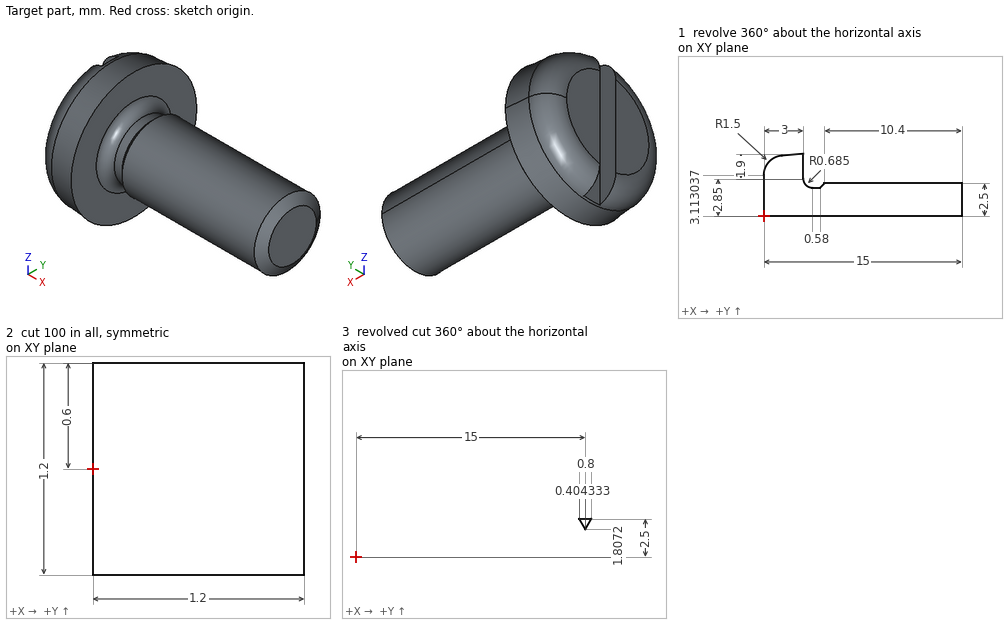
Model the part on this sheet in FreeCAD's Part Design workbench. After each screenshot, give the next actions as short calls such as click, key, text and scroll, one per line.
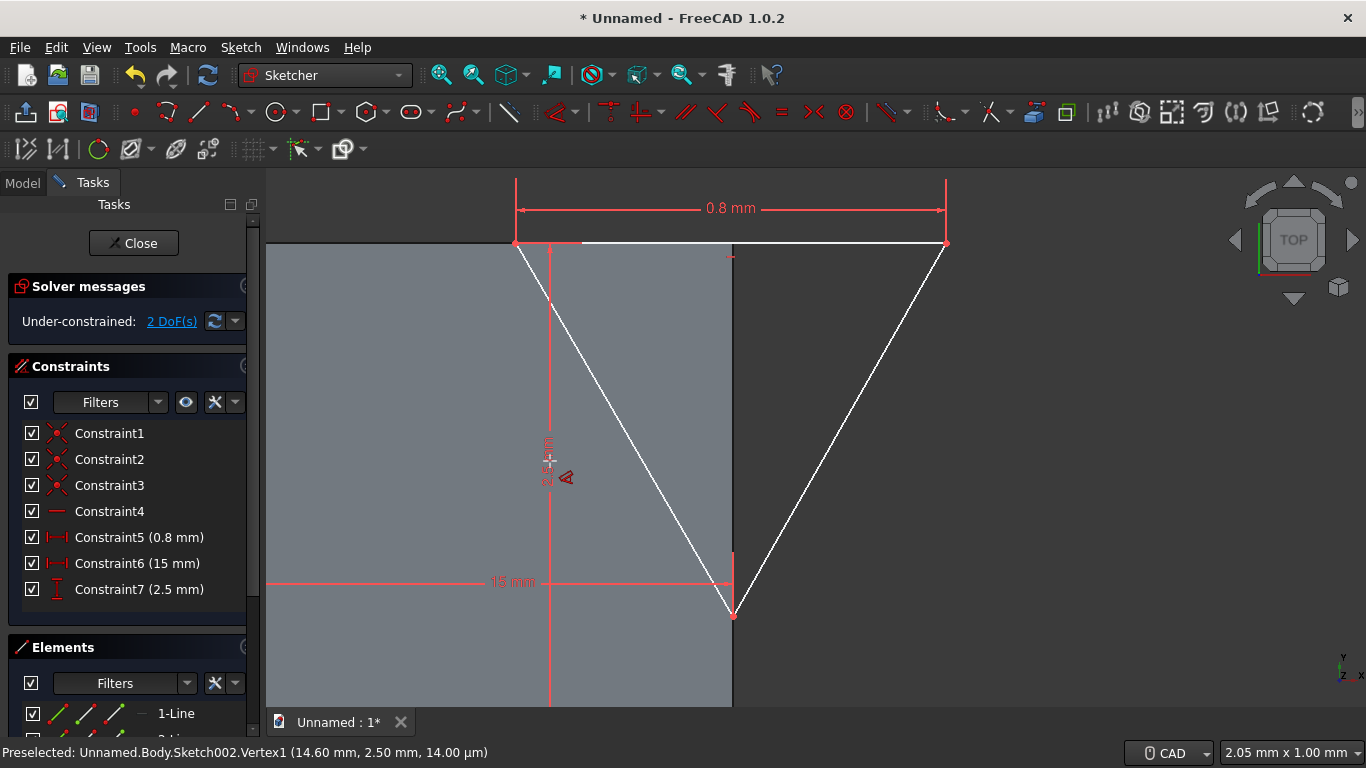
click(733, 617)
click(767, 648)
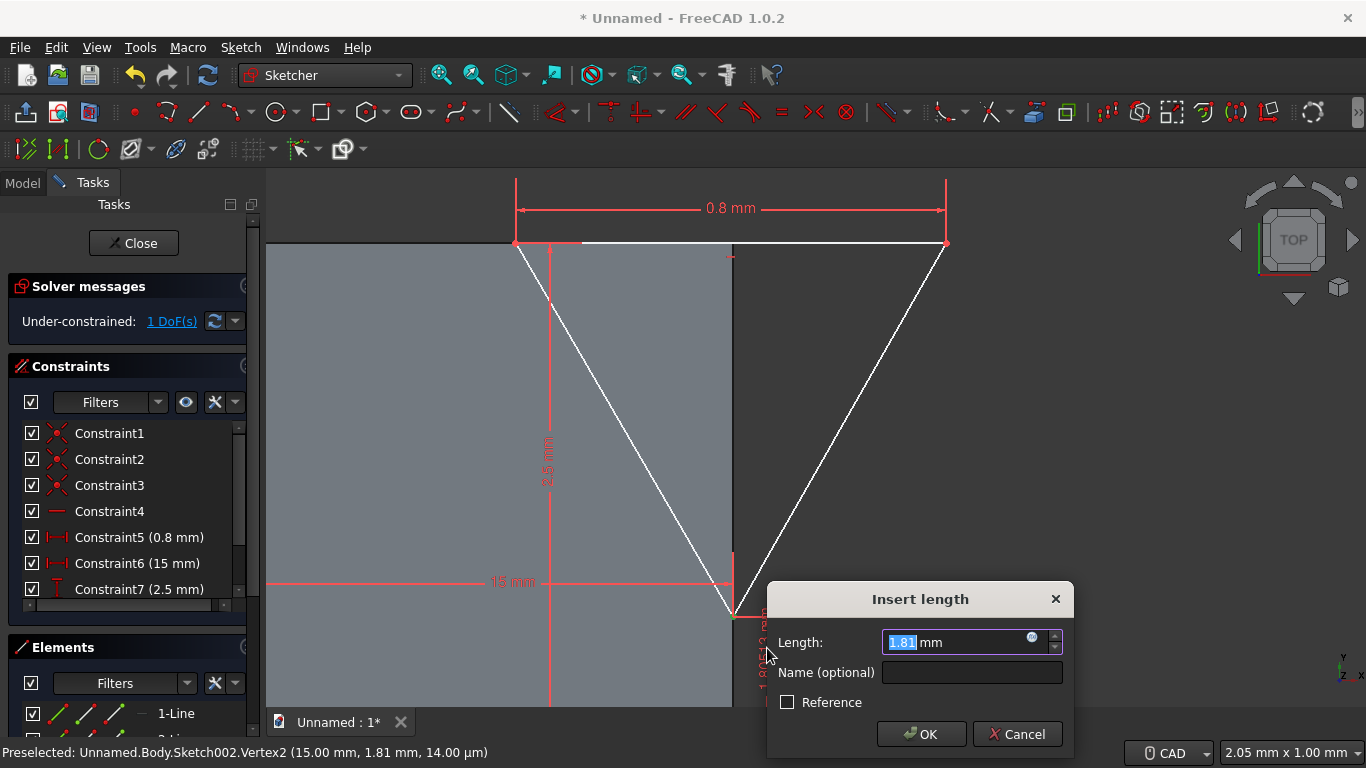
text(1.8072)
key(Return)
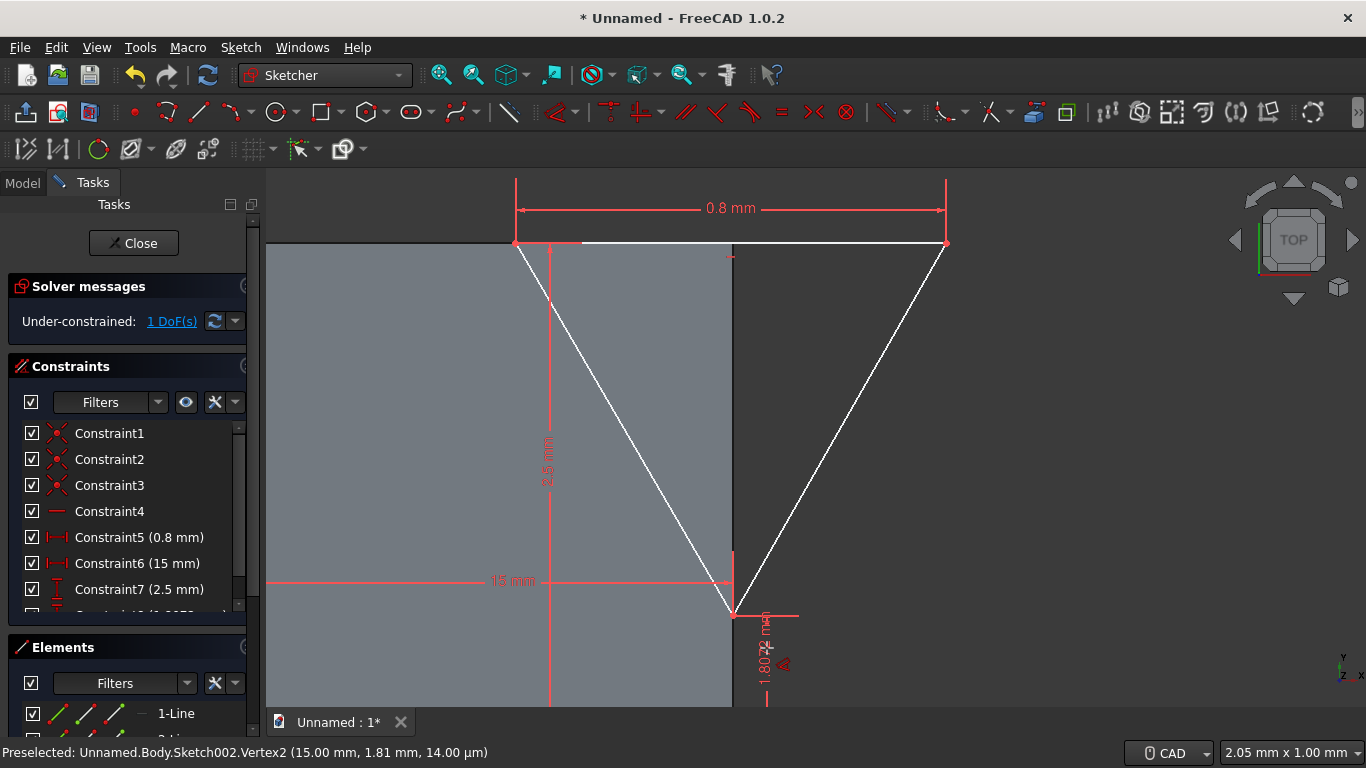
click(581, 355)
click(625, 209)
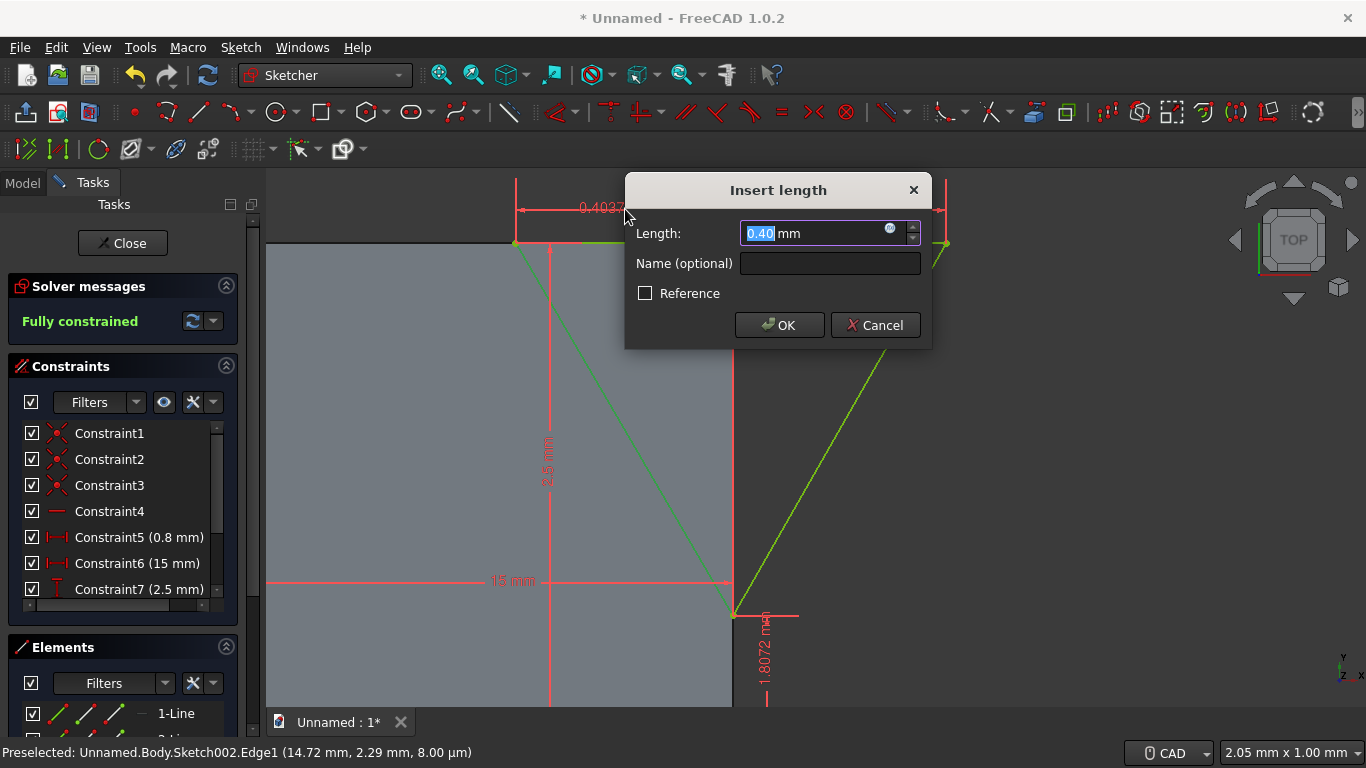
text(0.404333)
key(Return)
key(Escape)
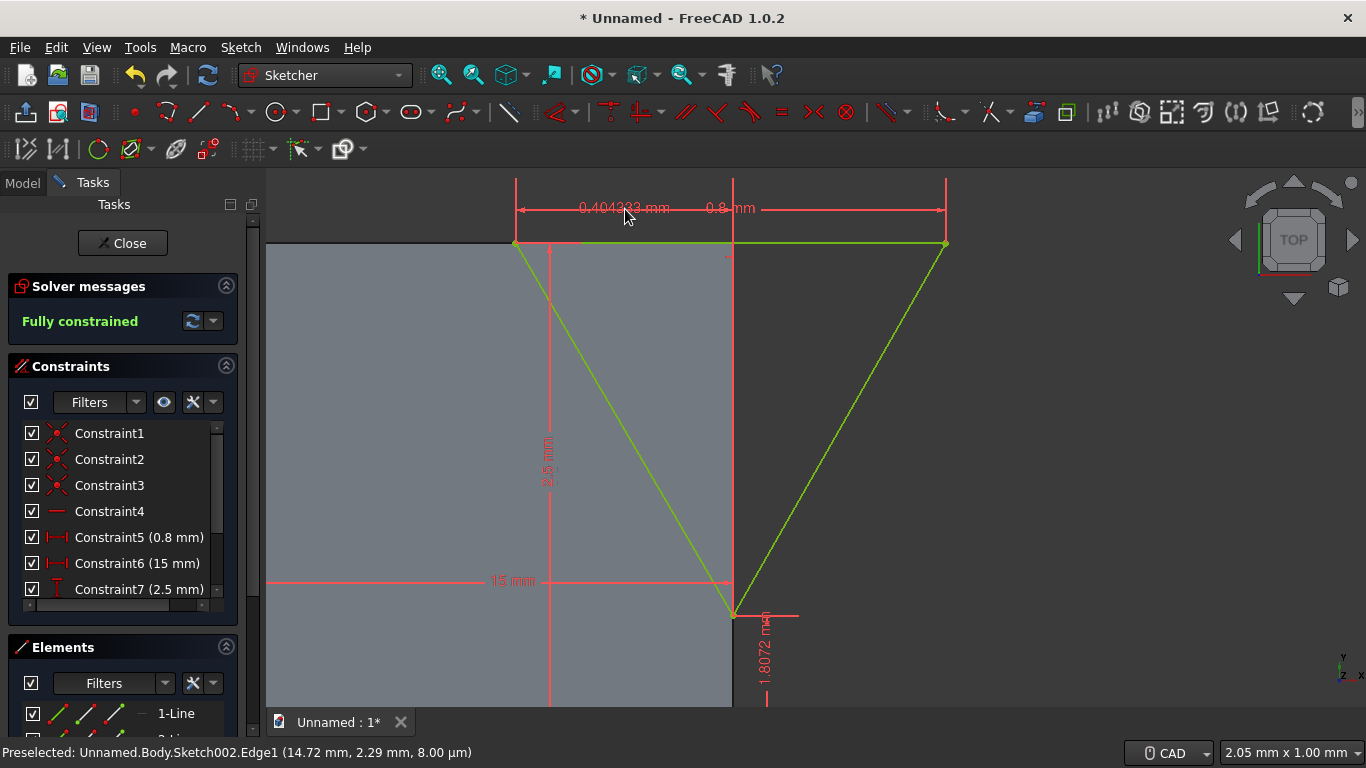
click(123, 243)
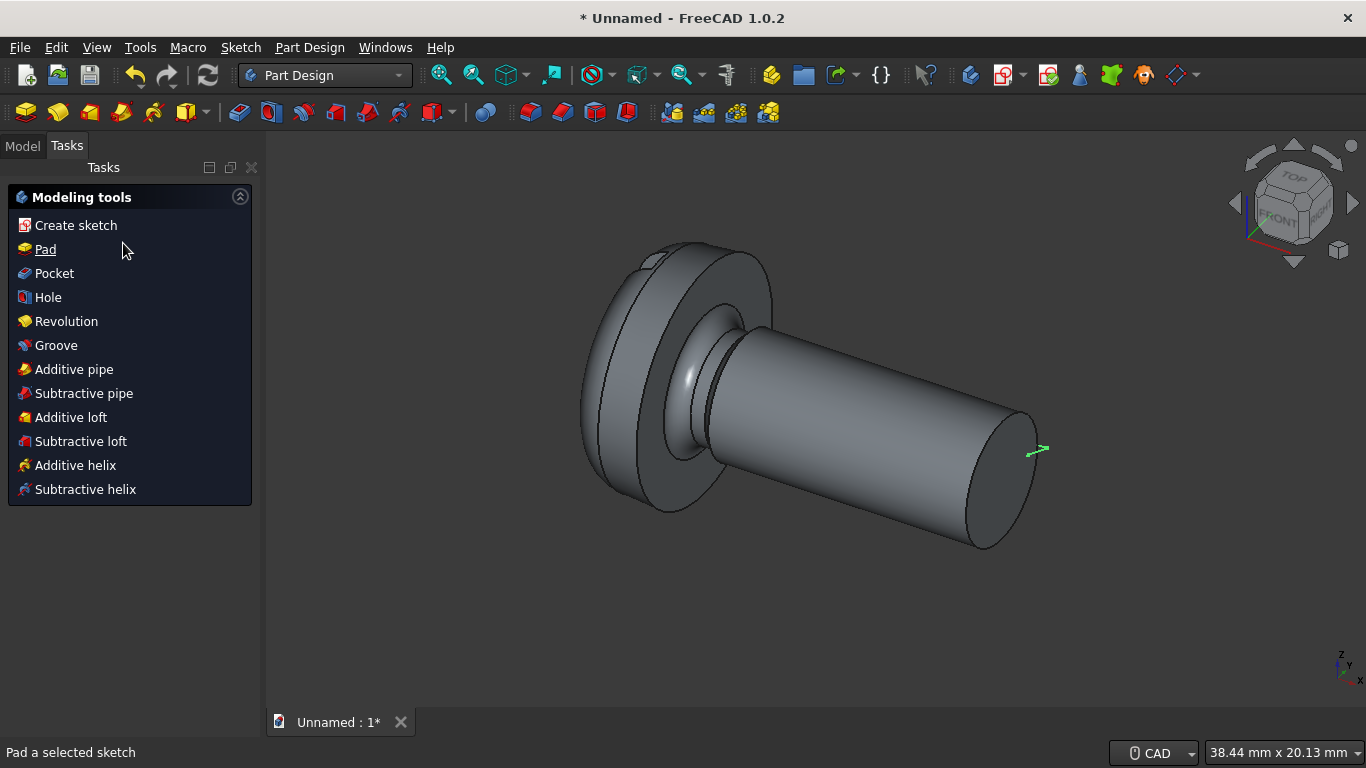
click(304, 112)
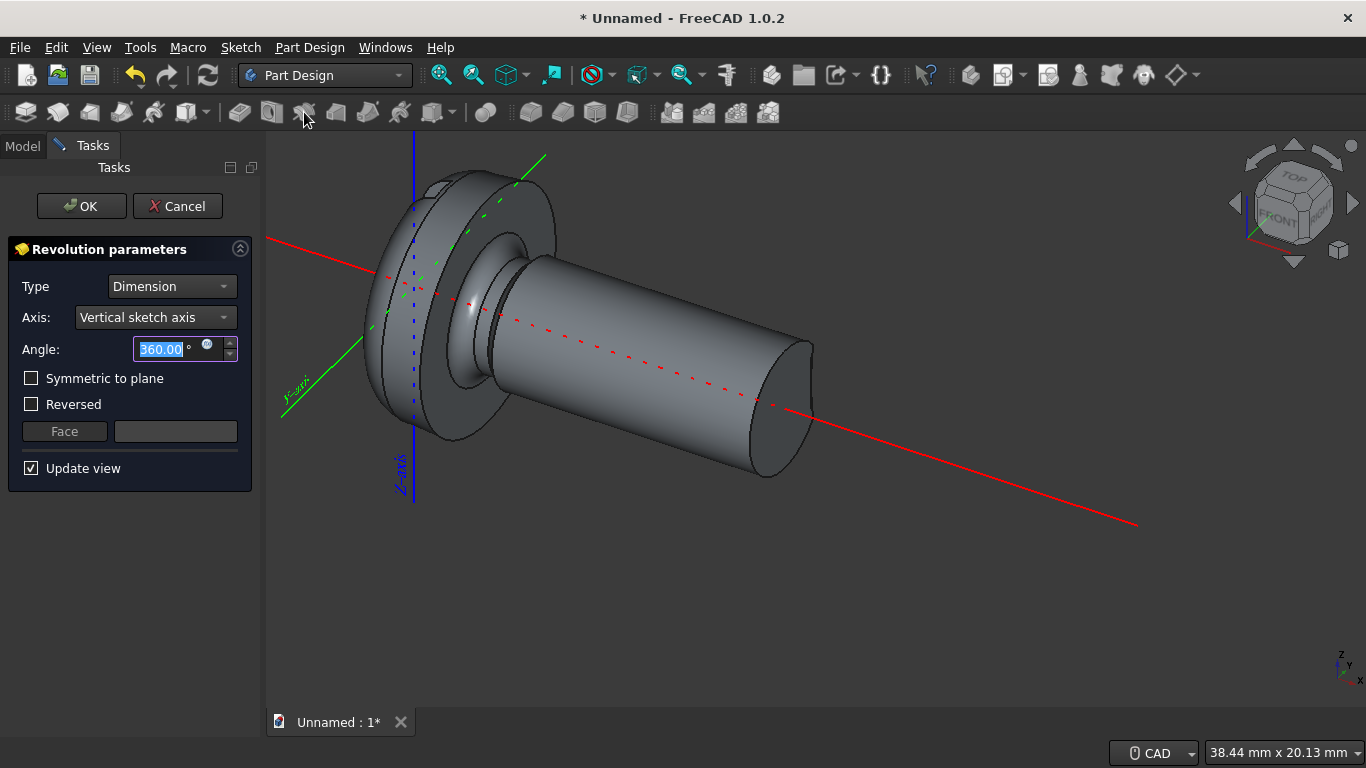
click(156, 318)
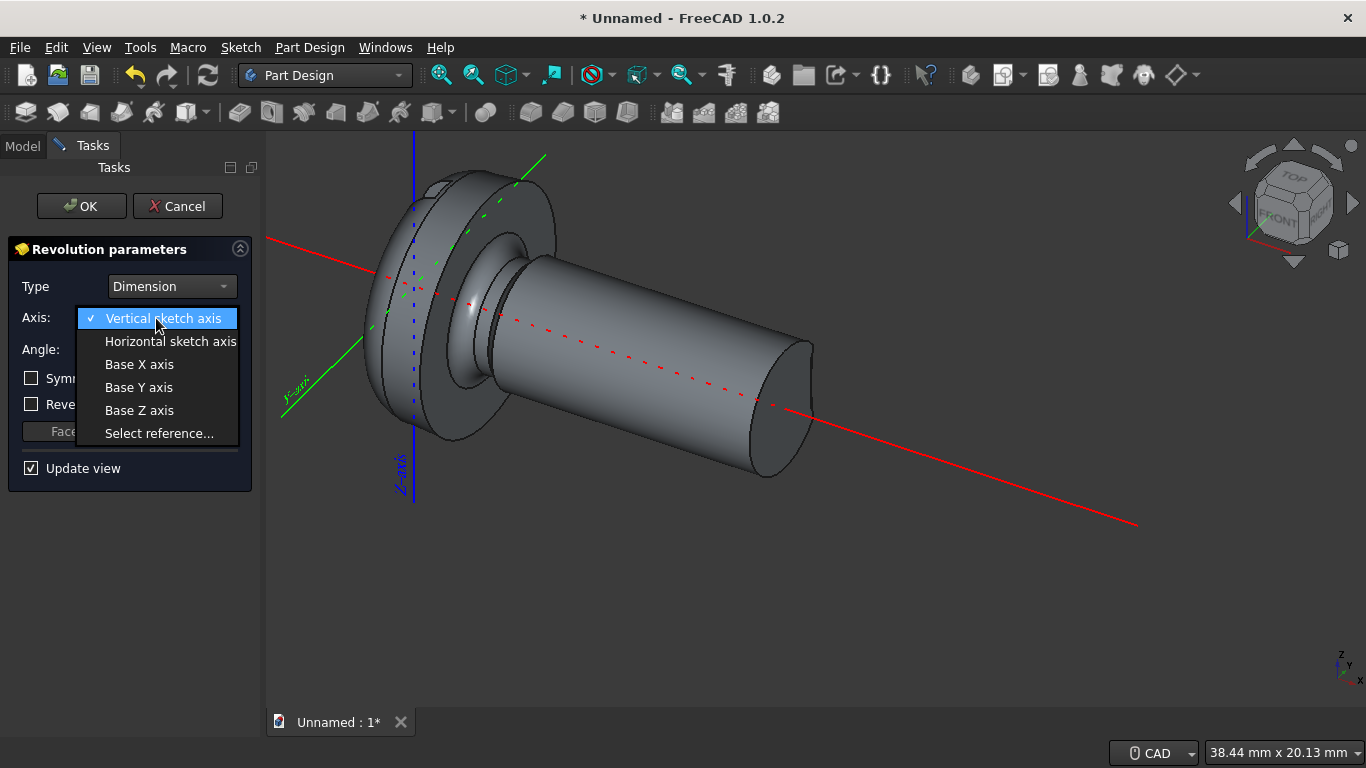
click(156, 342)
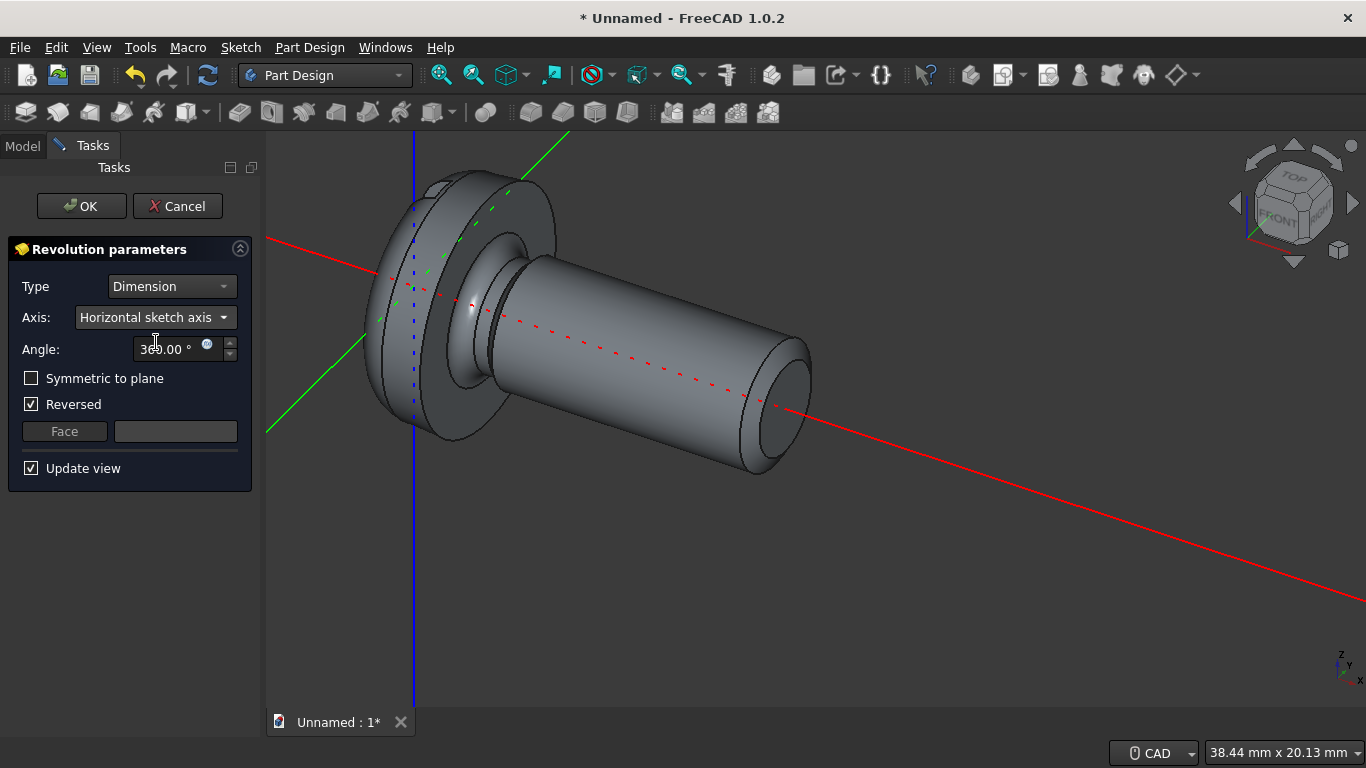
click(82, 206)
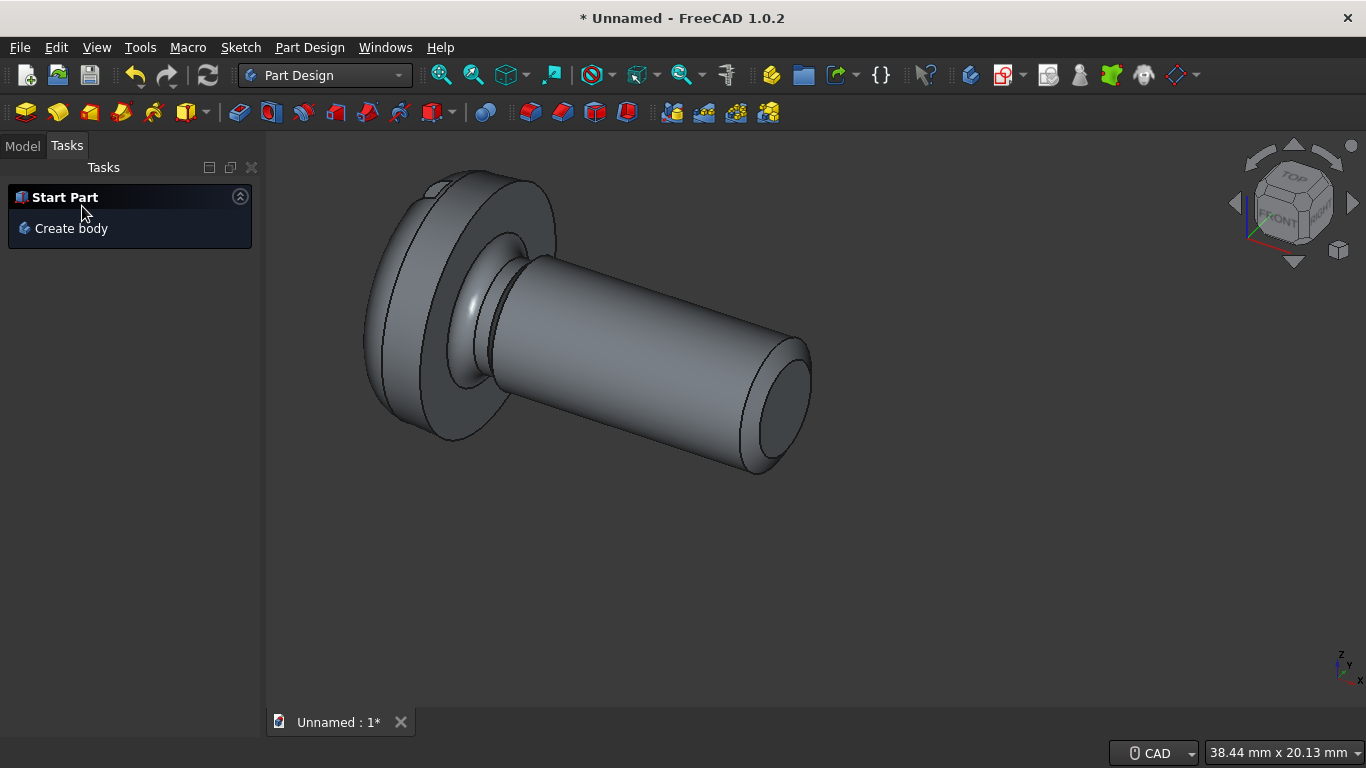
key(0)